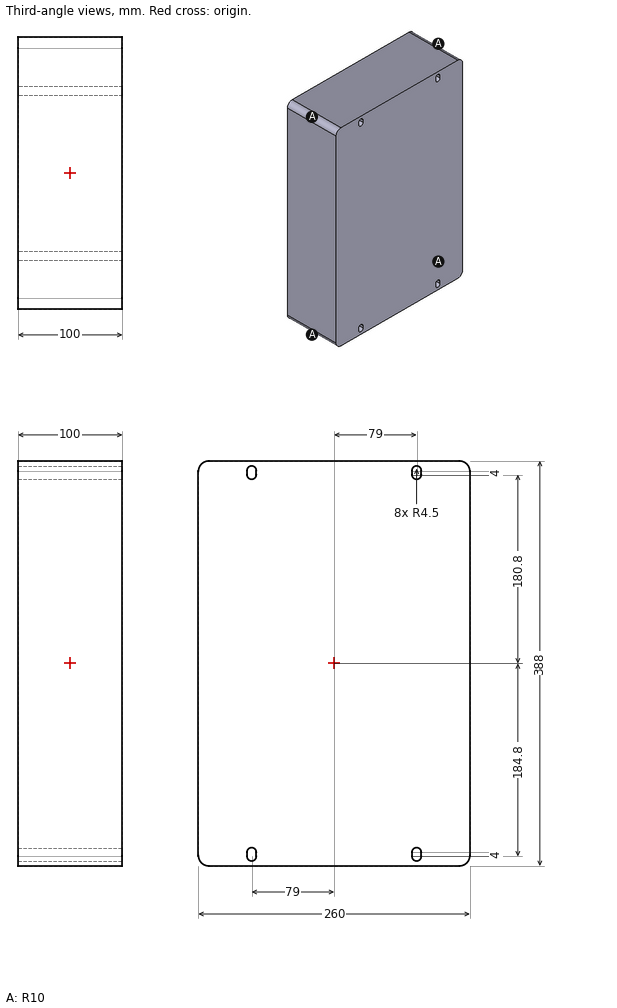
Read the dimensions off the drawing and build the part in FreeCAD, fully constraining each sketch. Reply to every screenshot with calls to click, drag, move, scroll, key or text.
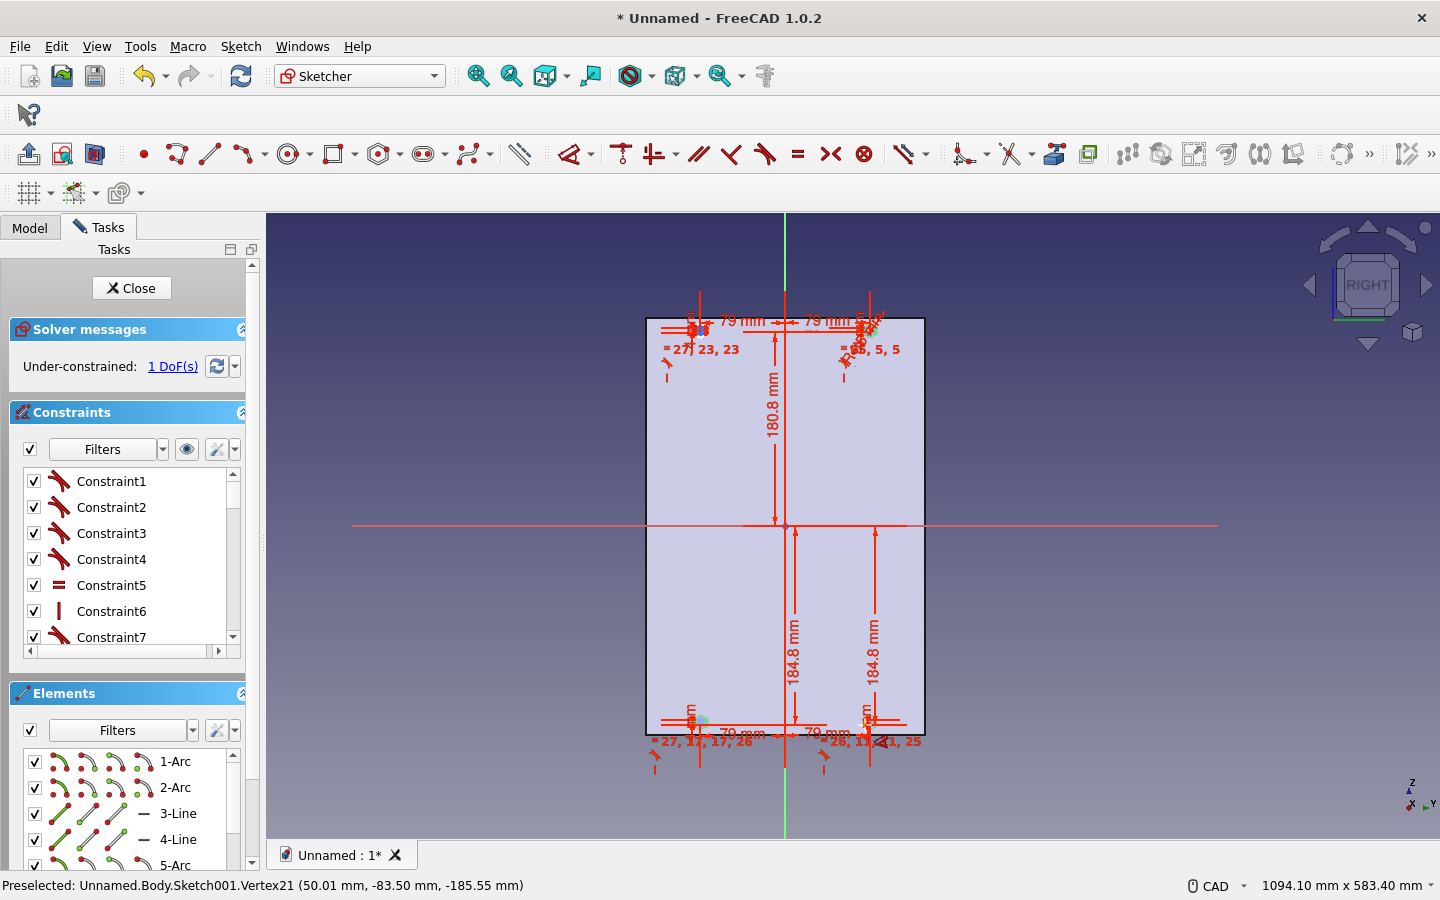
scroll(696, 333, up, 6)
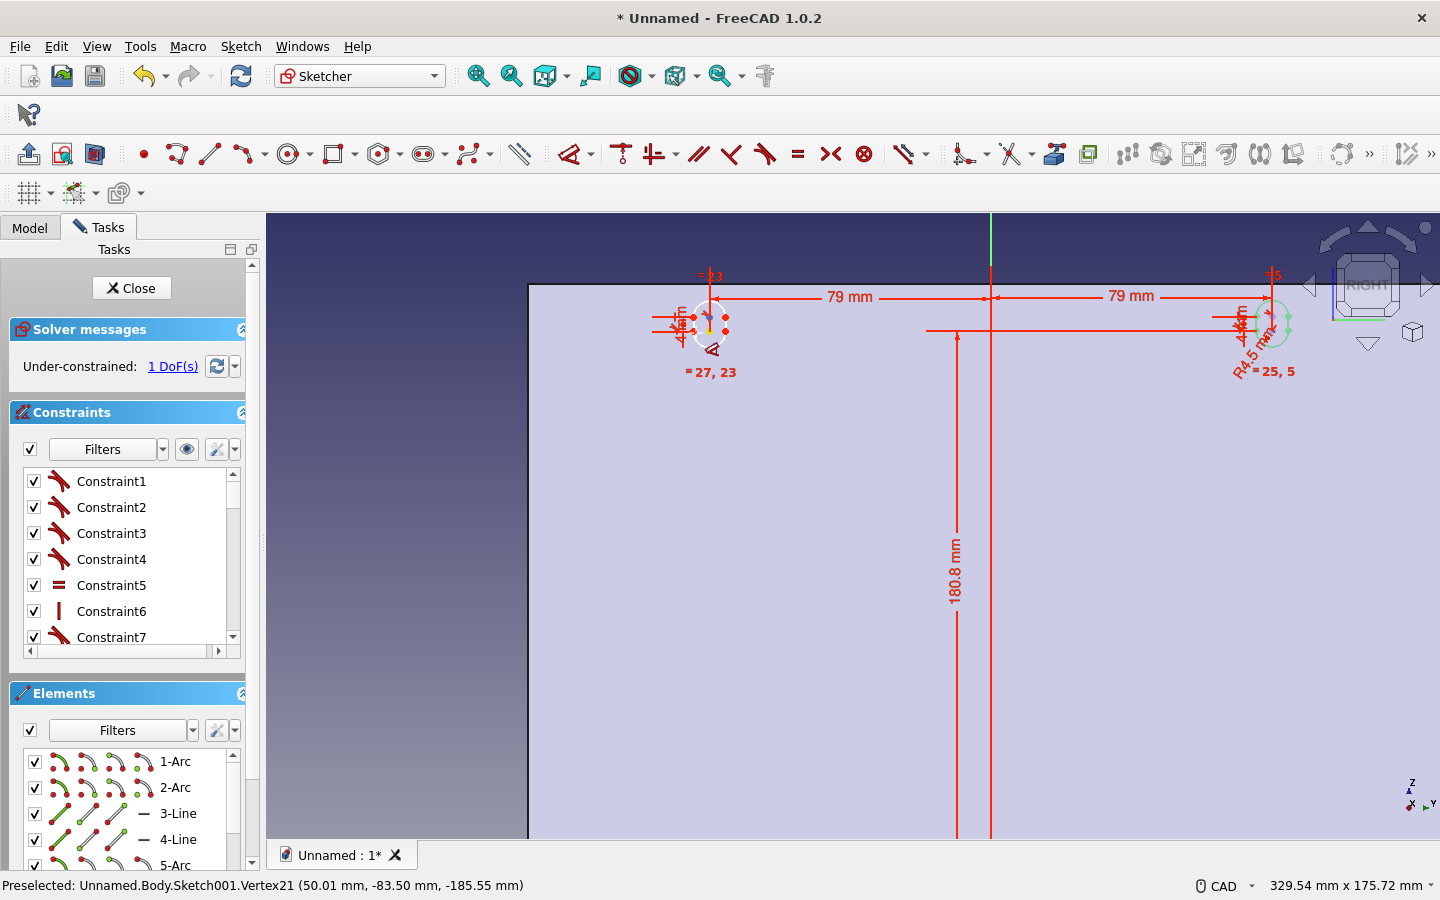
click(694, 332)
click(660, 571)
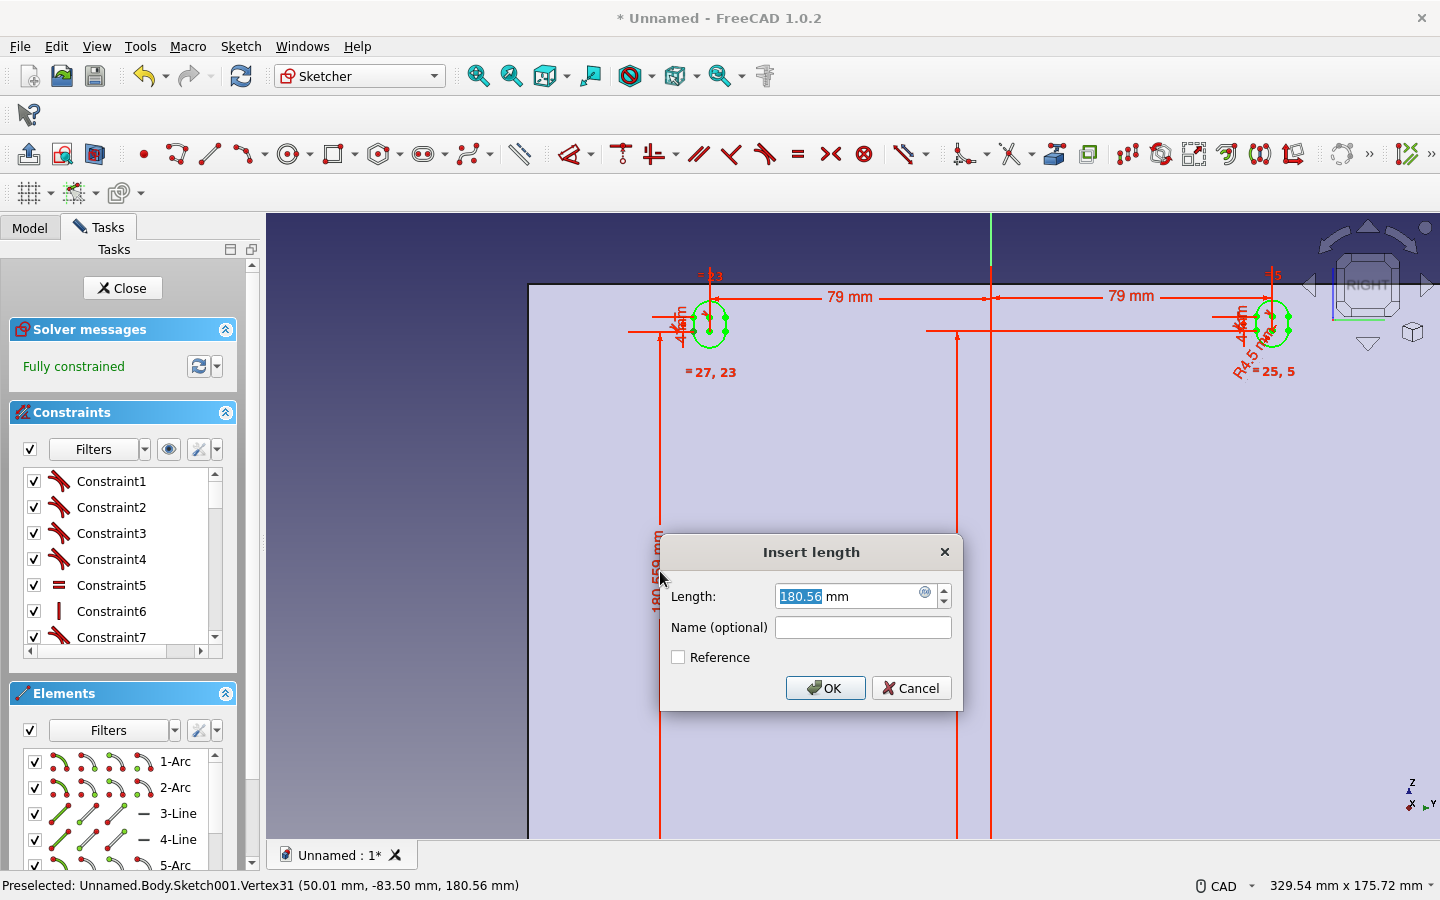
text(180.8)
key(Return)
key(Escape)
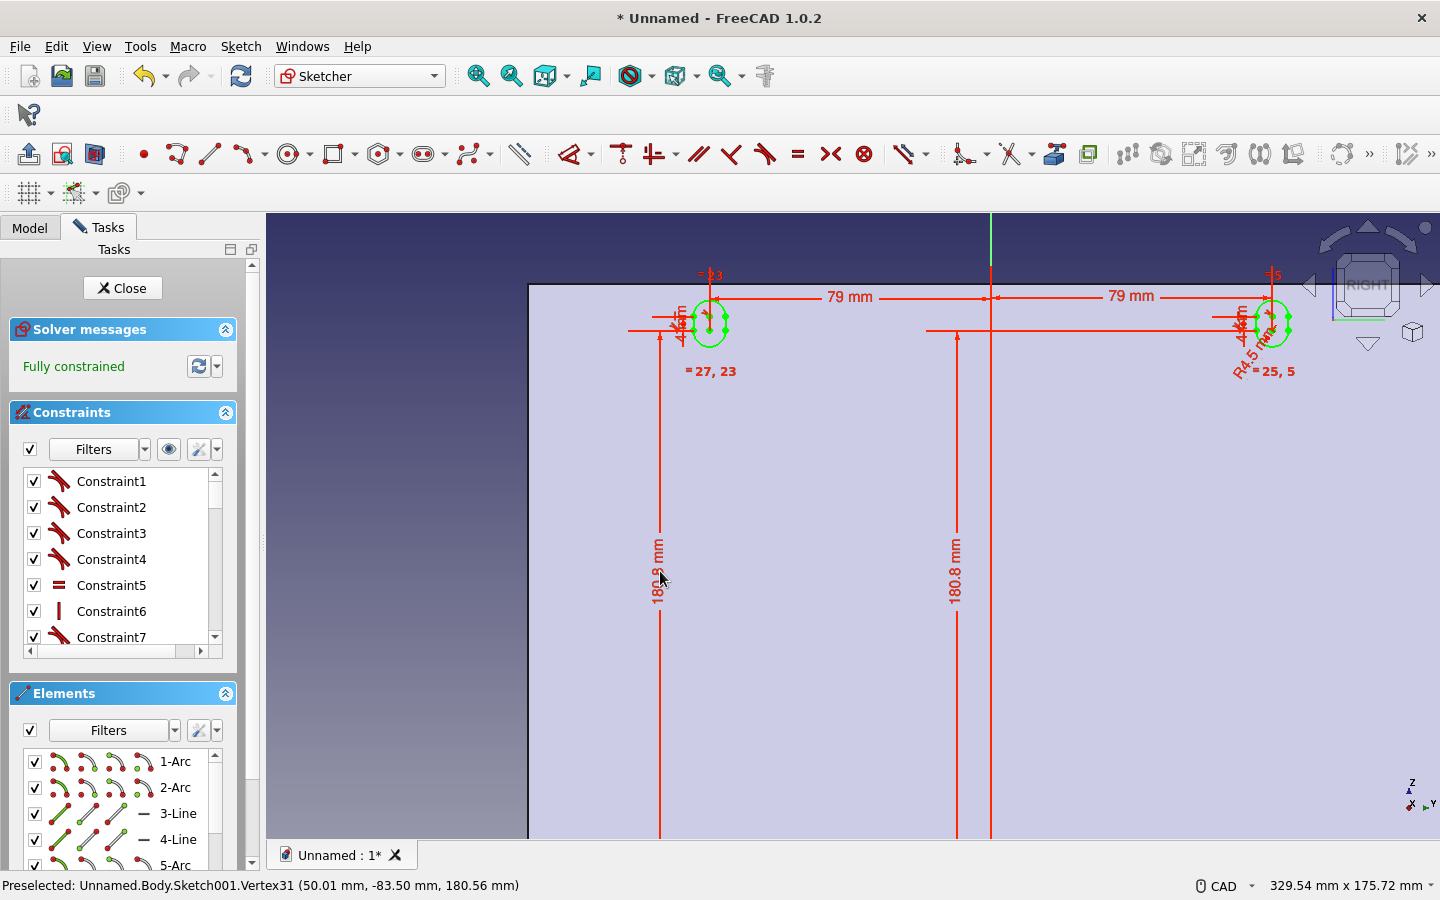
click(123, 288)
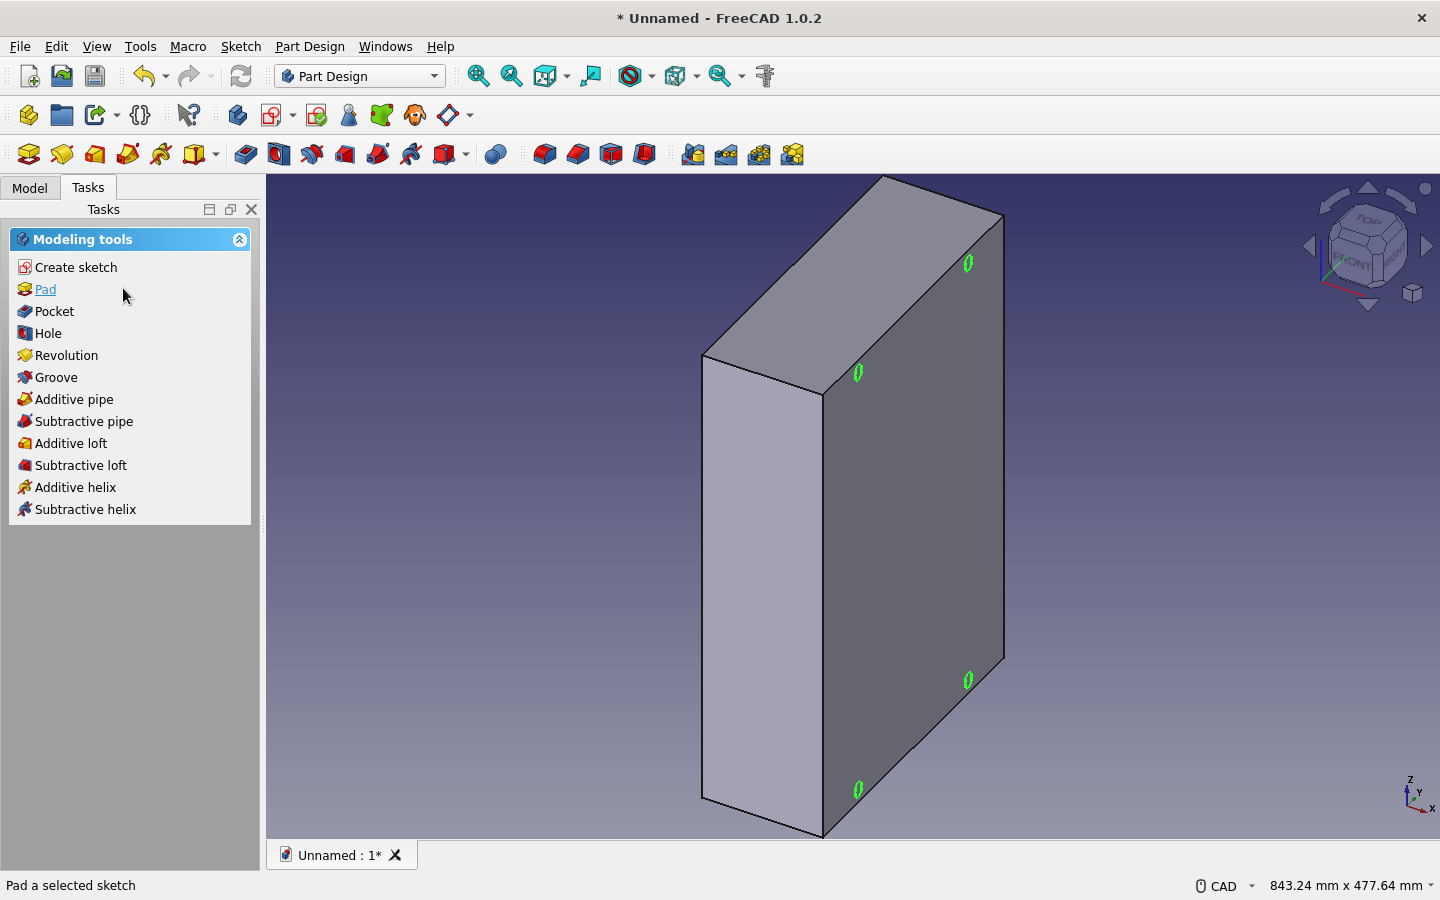
click(246, 154)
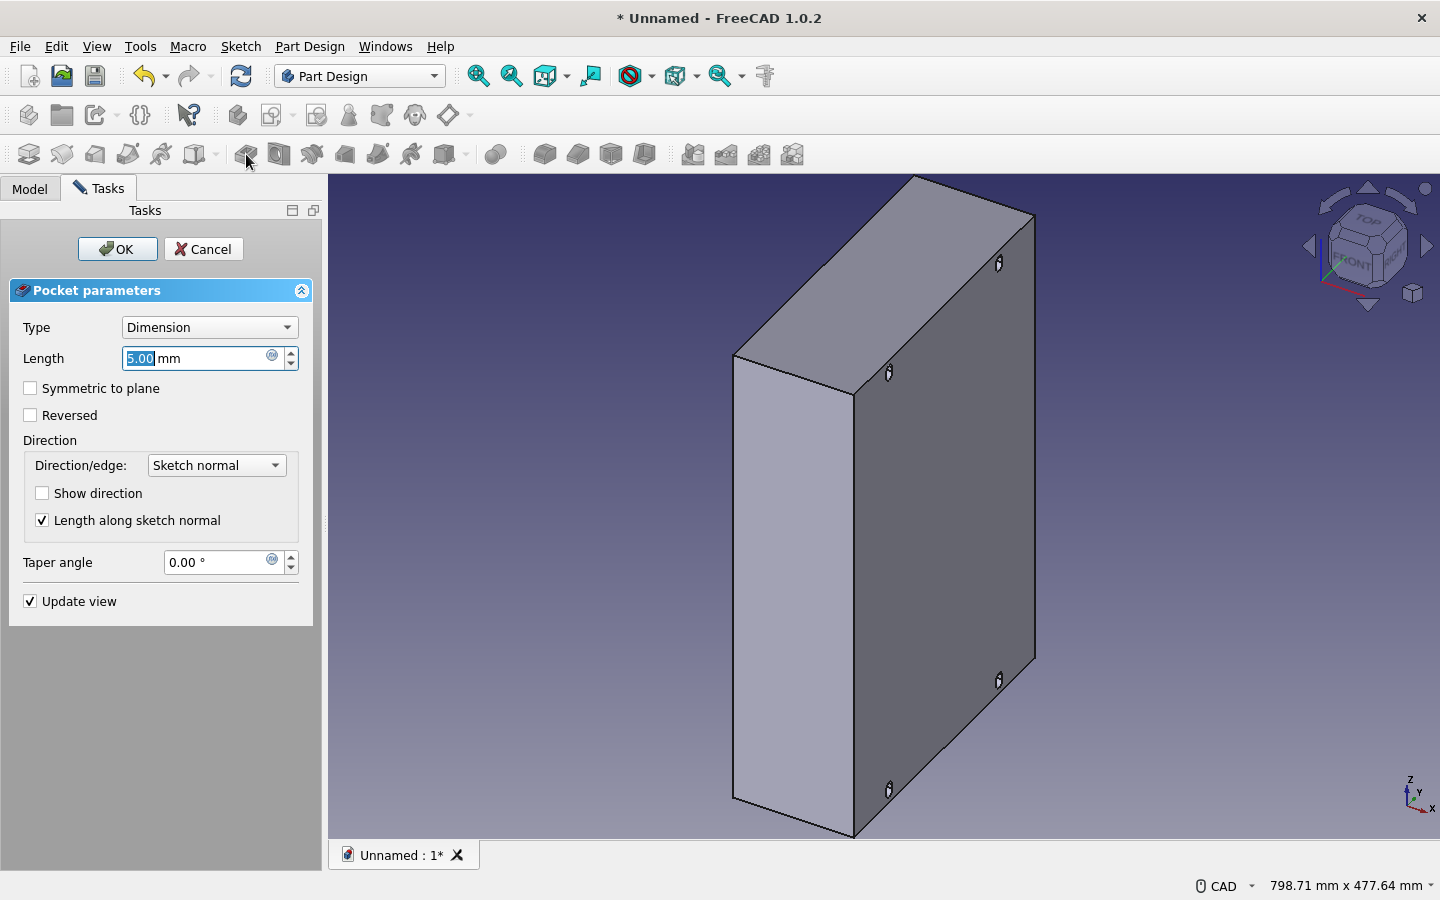
text(100)
key(Tab)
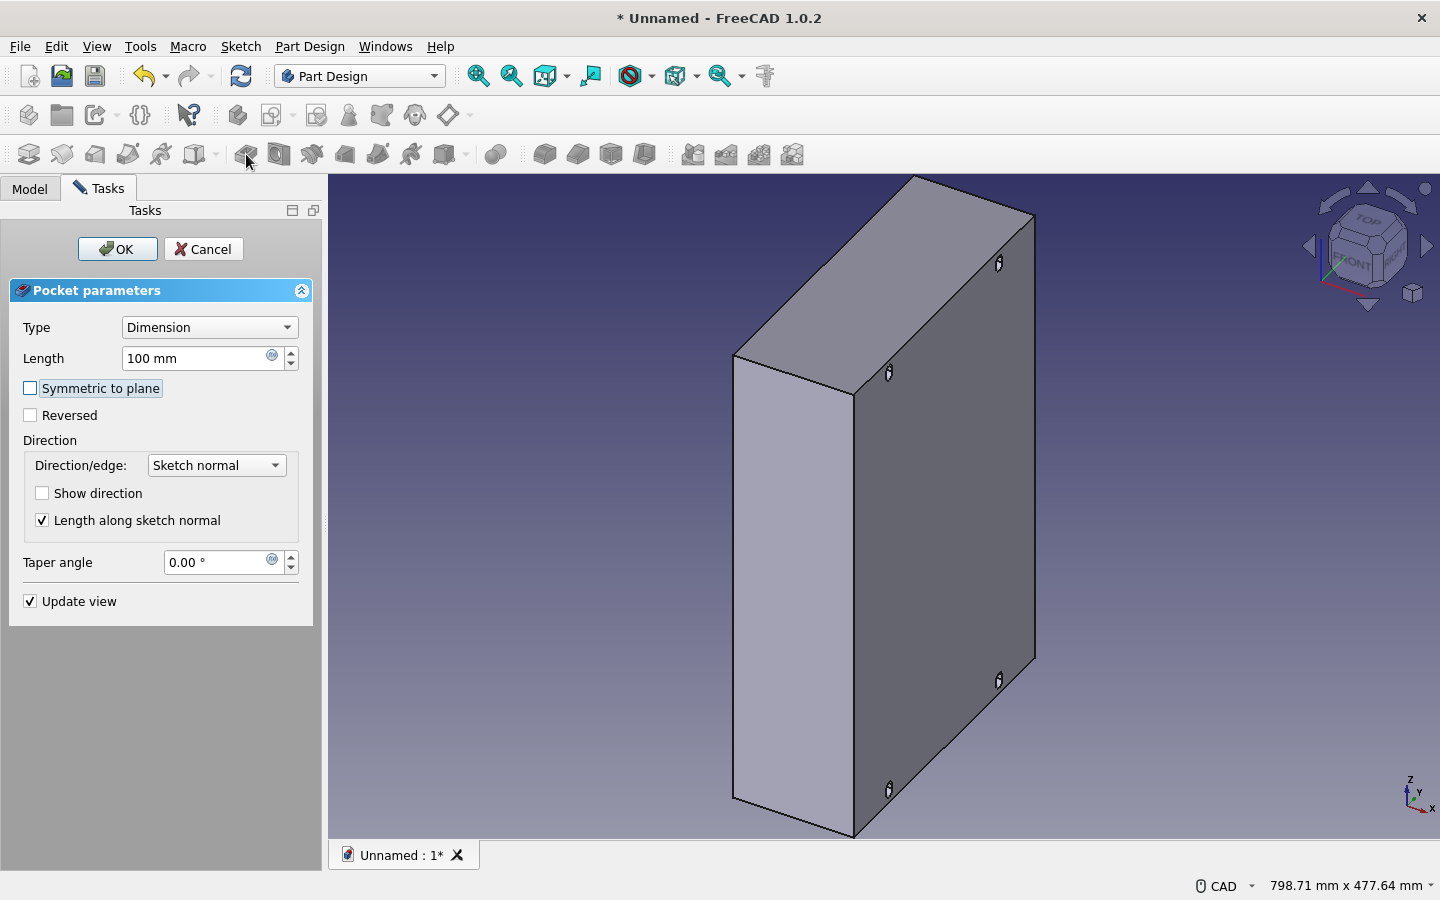
click(118, 249)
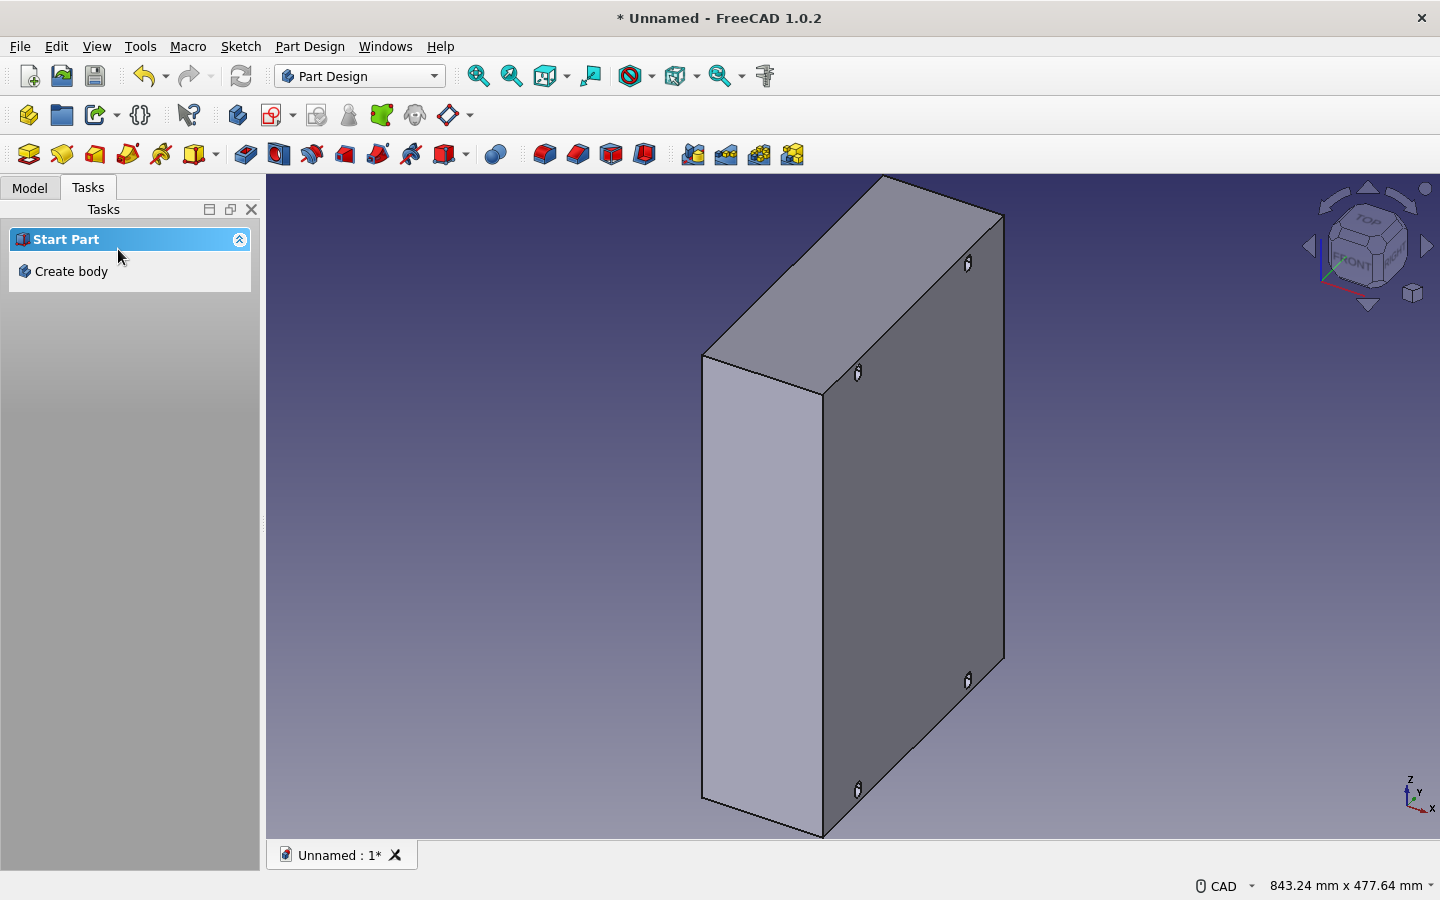
click(763, 374)